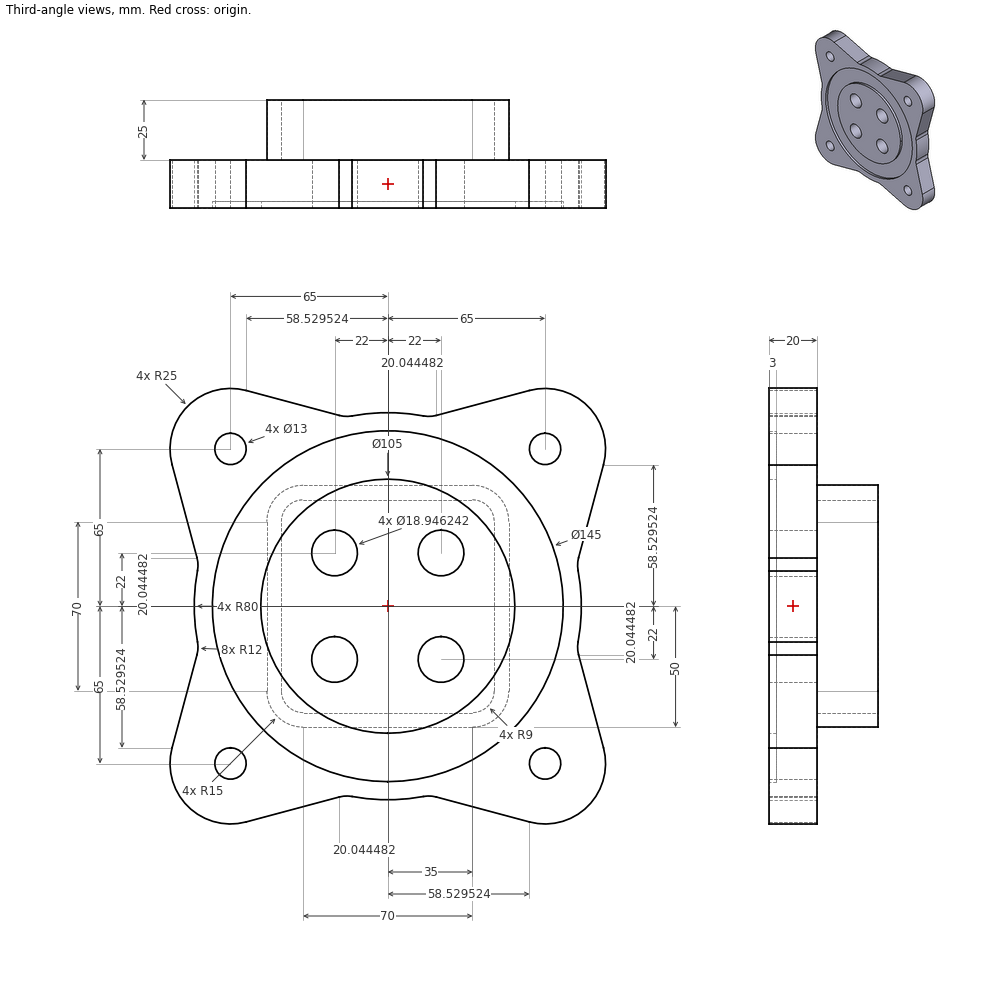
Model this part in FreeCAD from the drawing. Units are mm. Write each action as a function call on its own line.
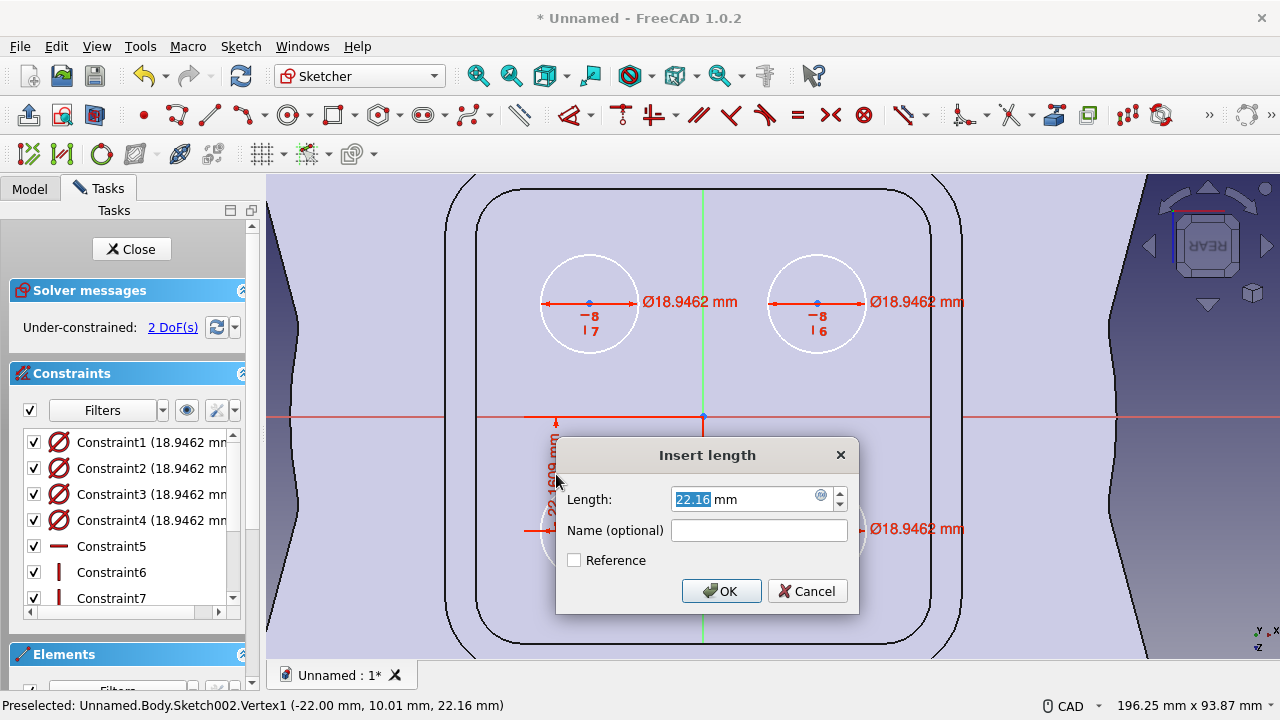
text(22)
key(Return)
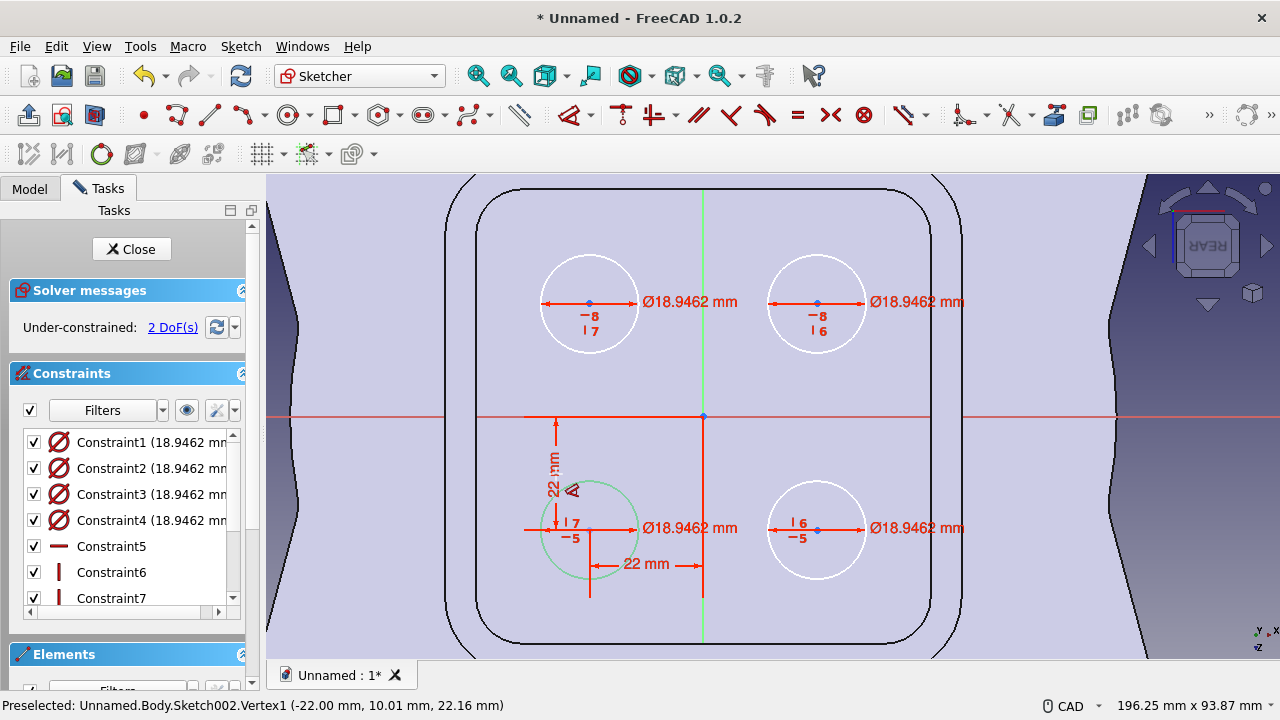
click(817, 530)
click(760, 564)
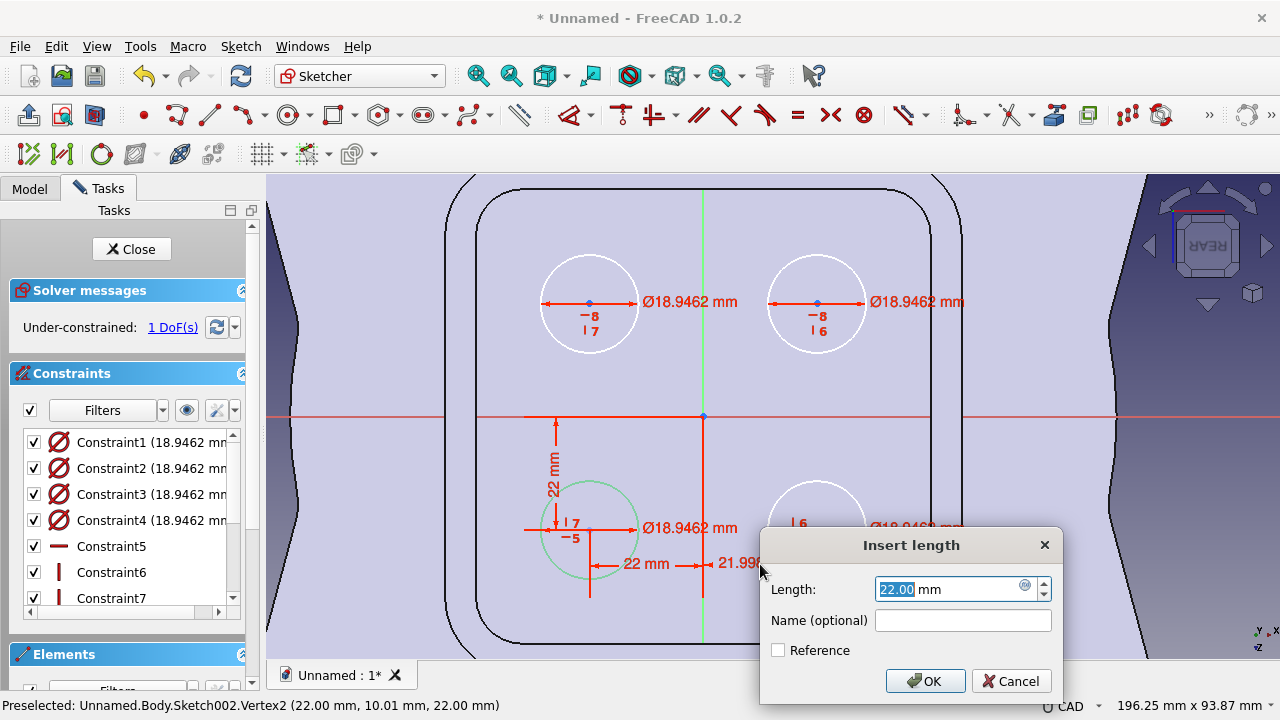
text(22)
key(Return)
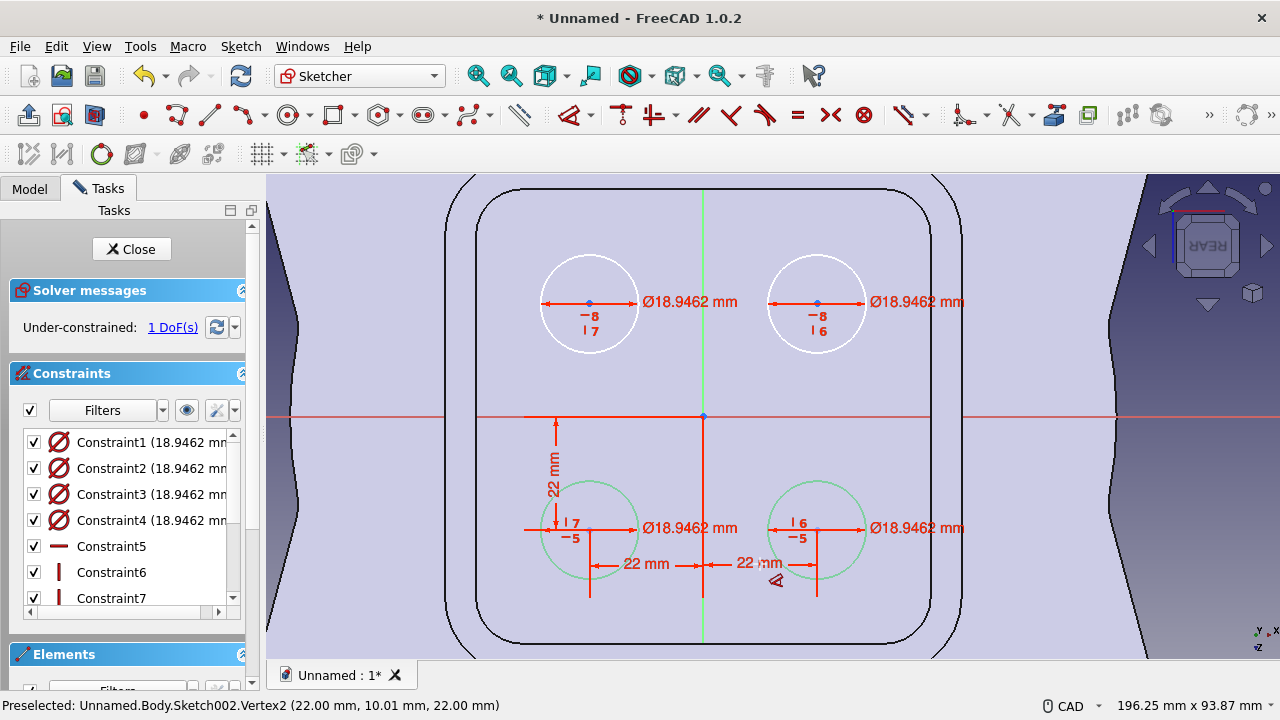
click(817, 304)
click(851, 360)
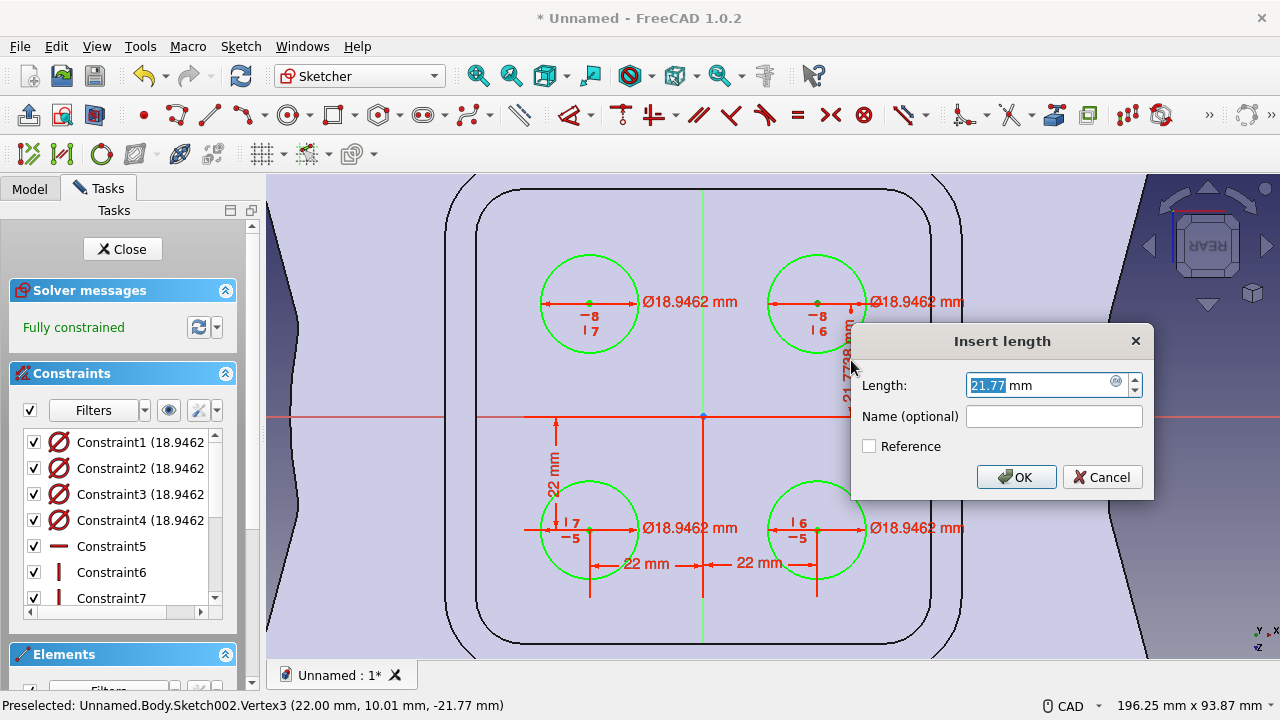
text(22)
key(Return)
key(Escape)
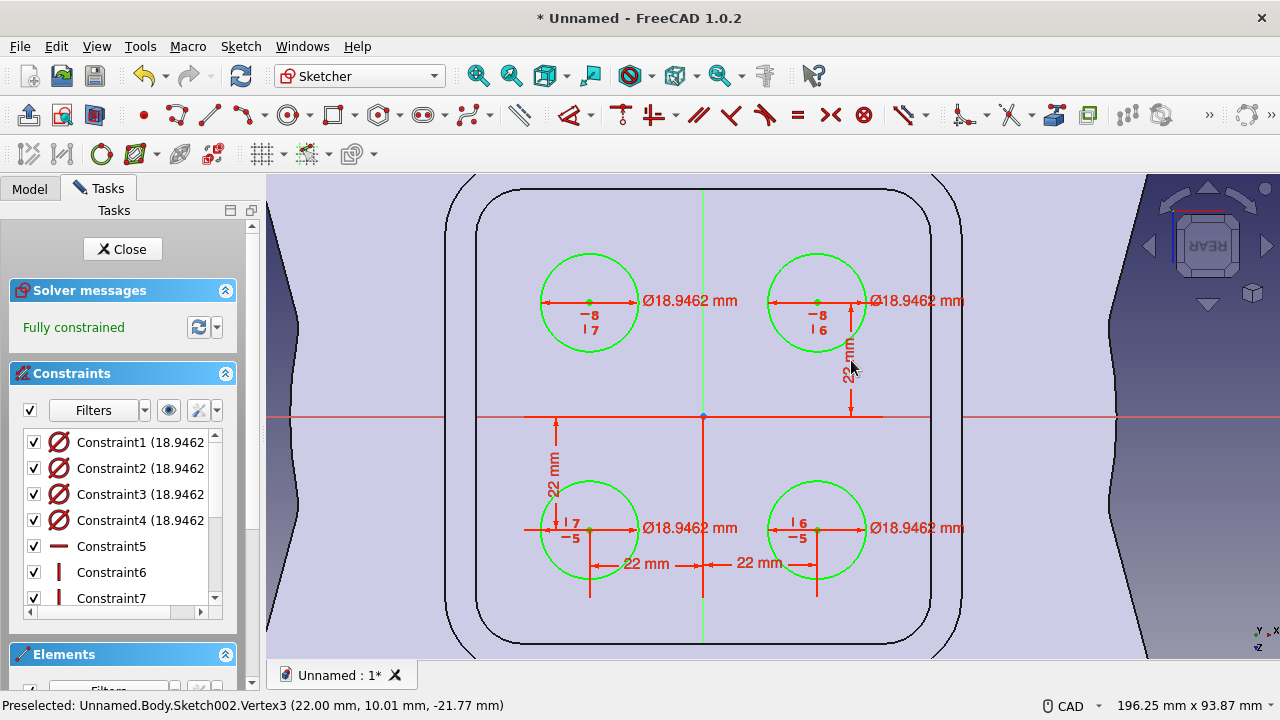
click(123, 249)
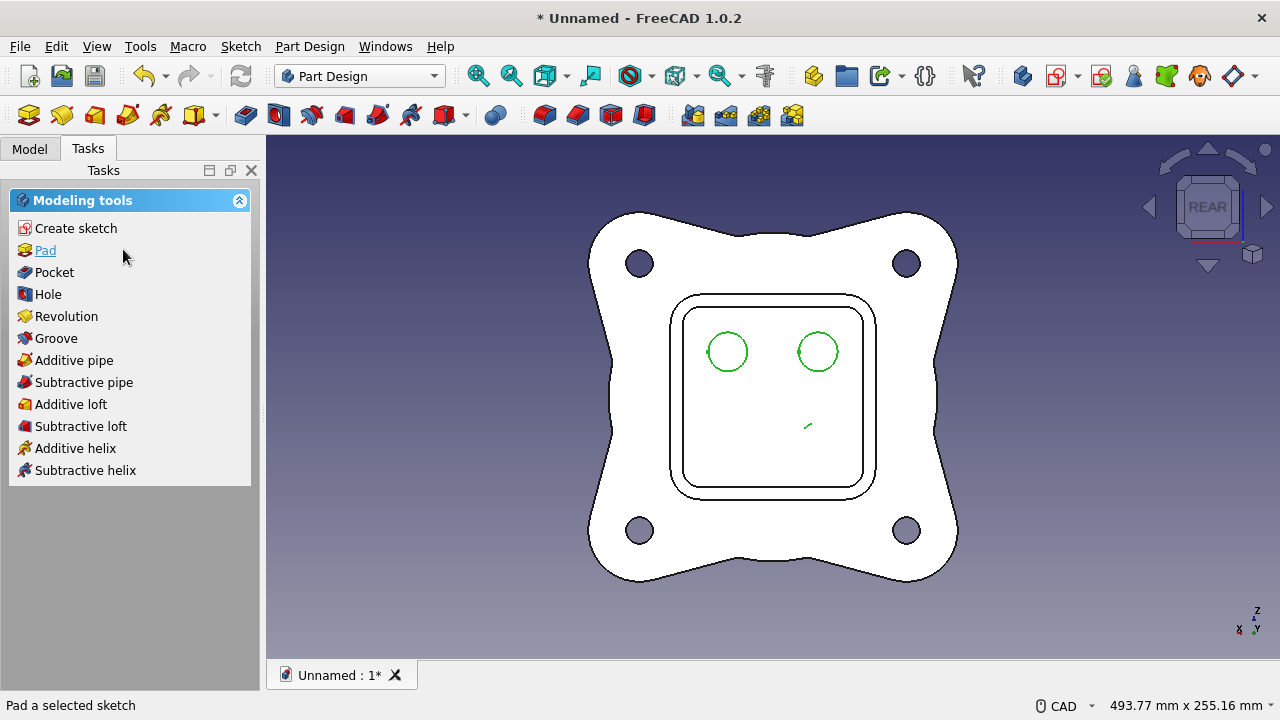
click(246, 116)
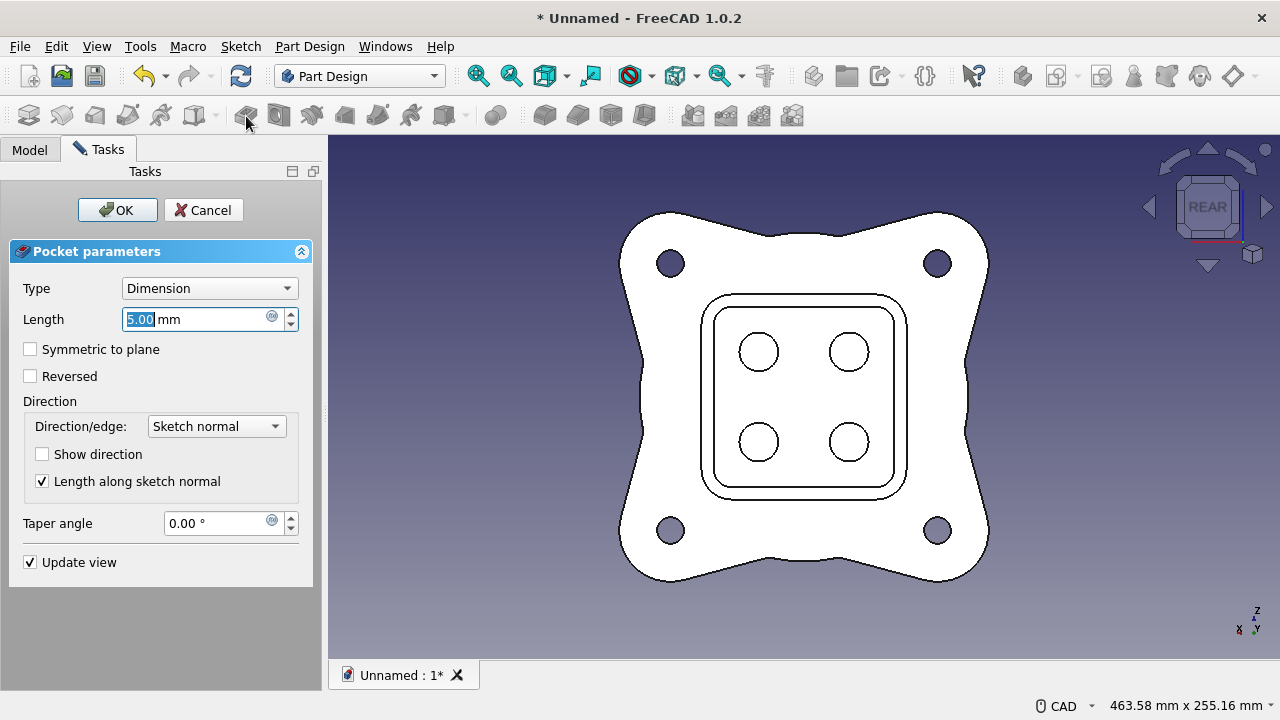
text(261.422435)
key(Tab)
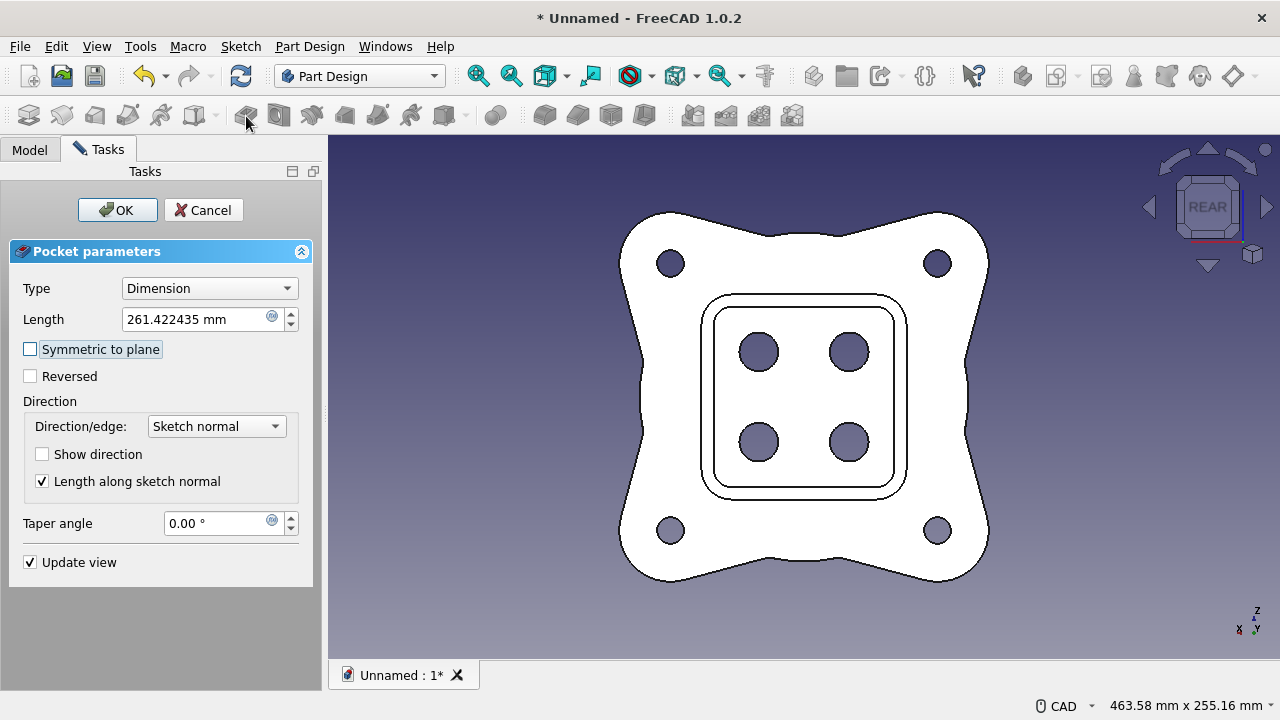
click(31, 349)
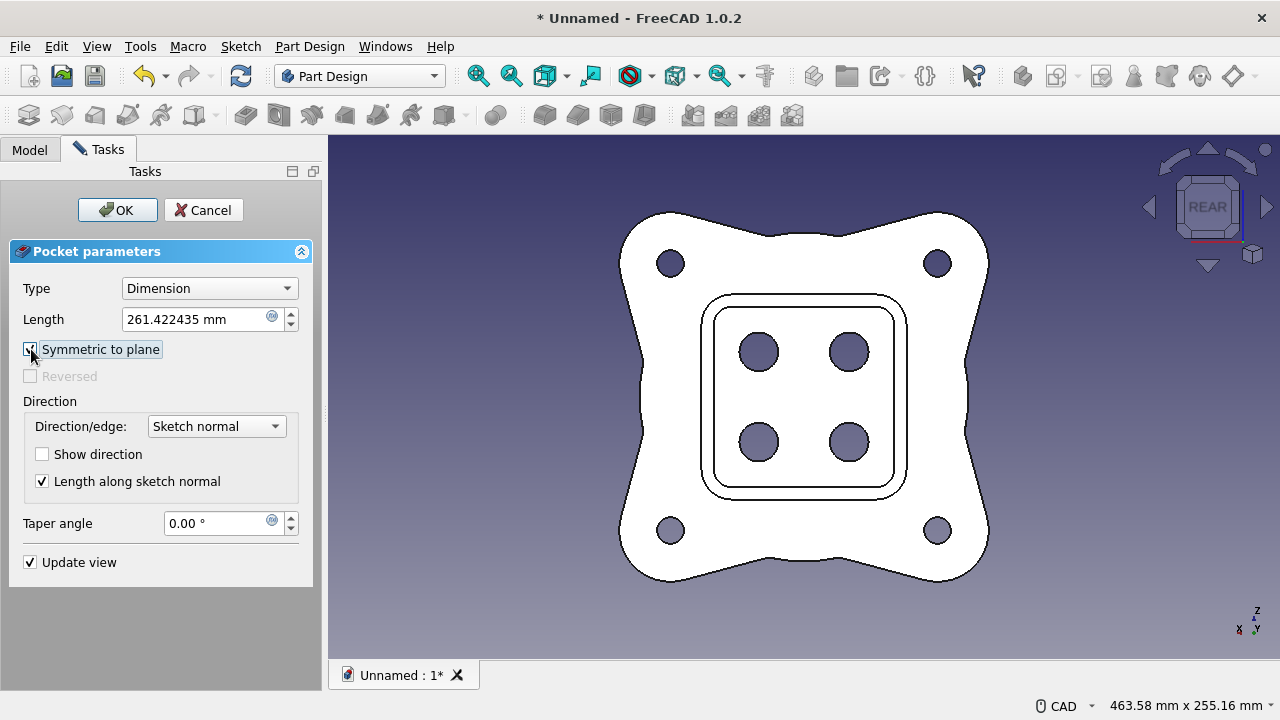
click(118, 210)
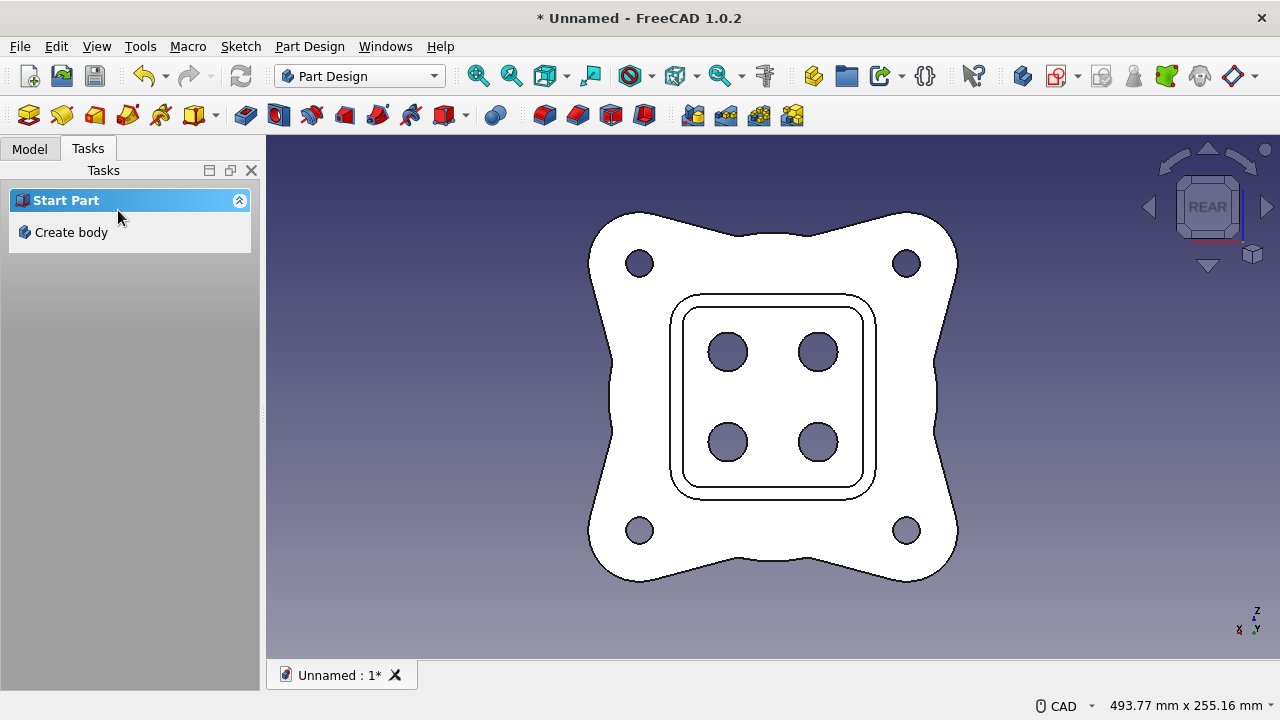
key(0)